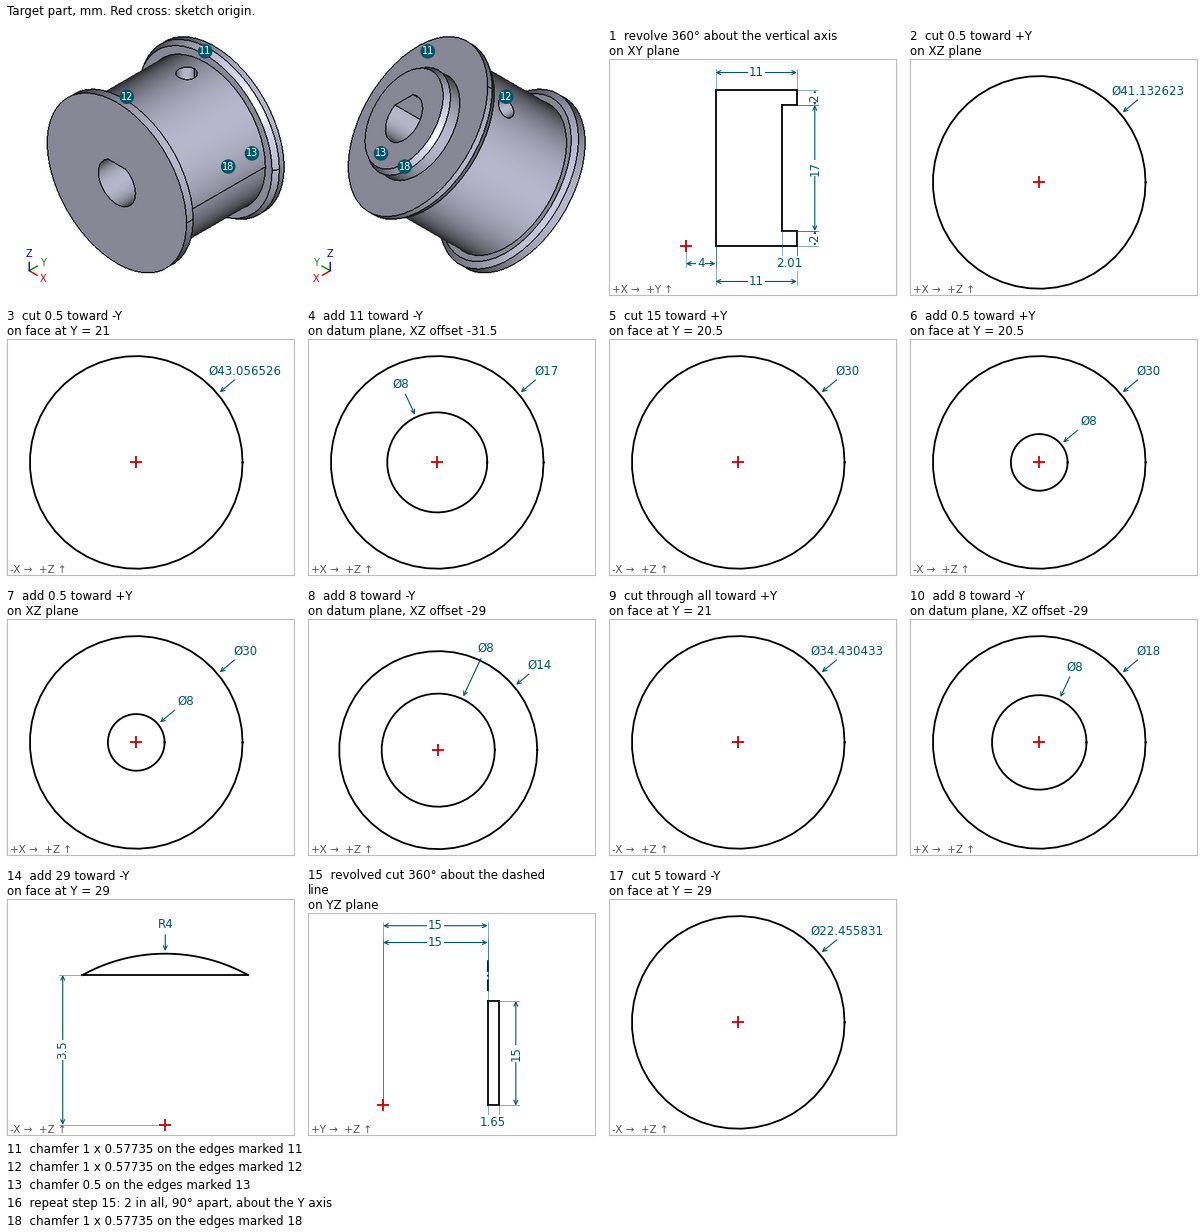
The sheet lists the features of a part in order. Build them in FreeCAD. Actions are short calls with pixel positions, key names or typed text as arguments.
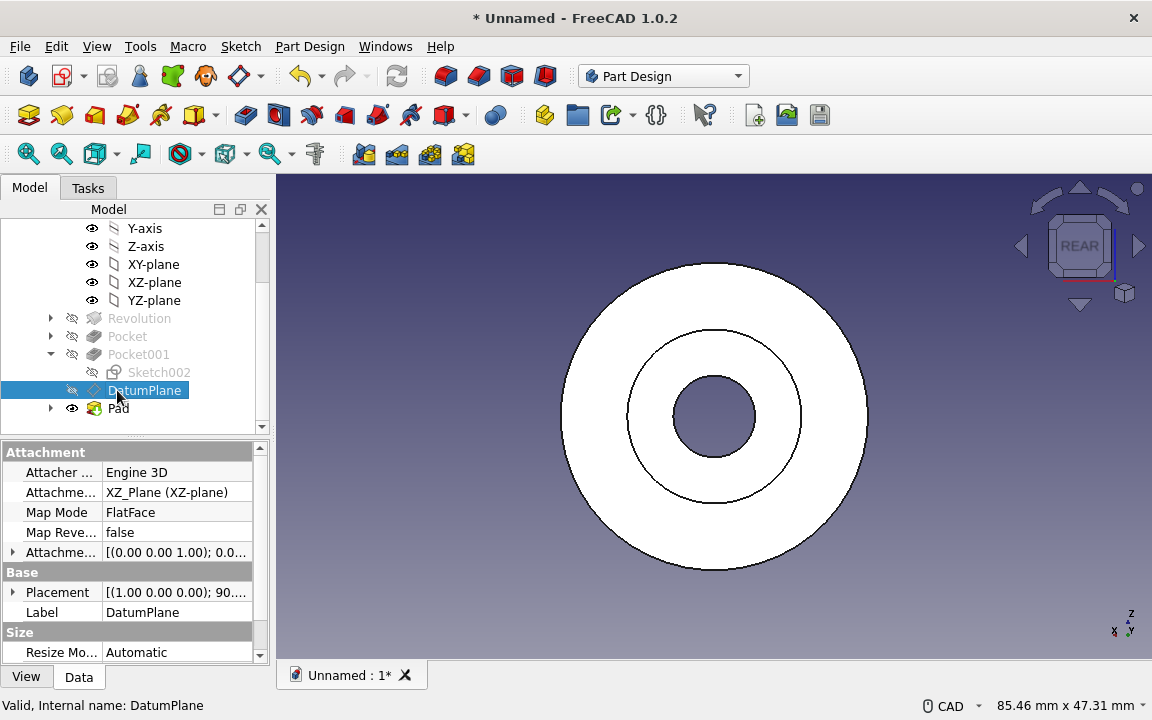
click(802, 328)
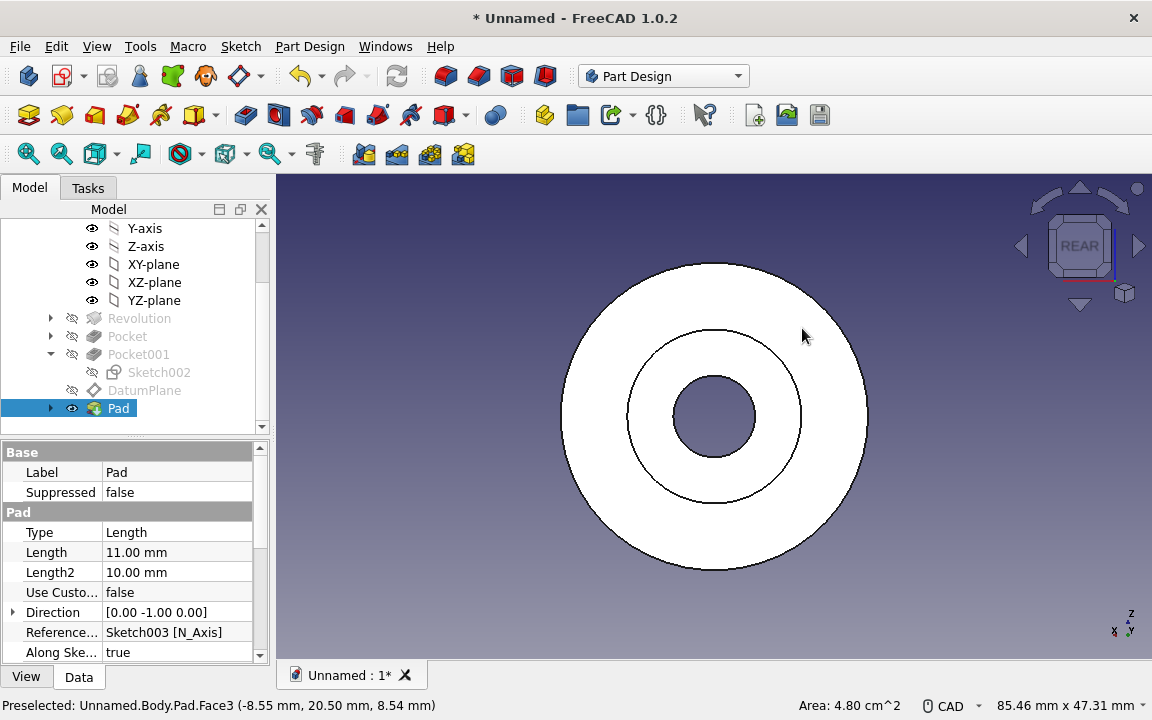
click(62, 76)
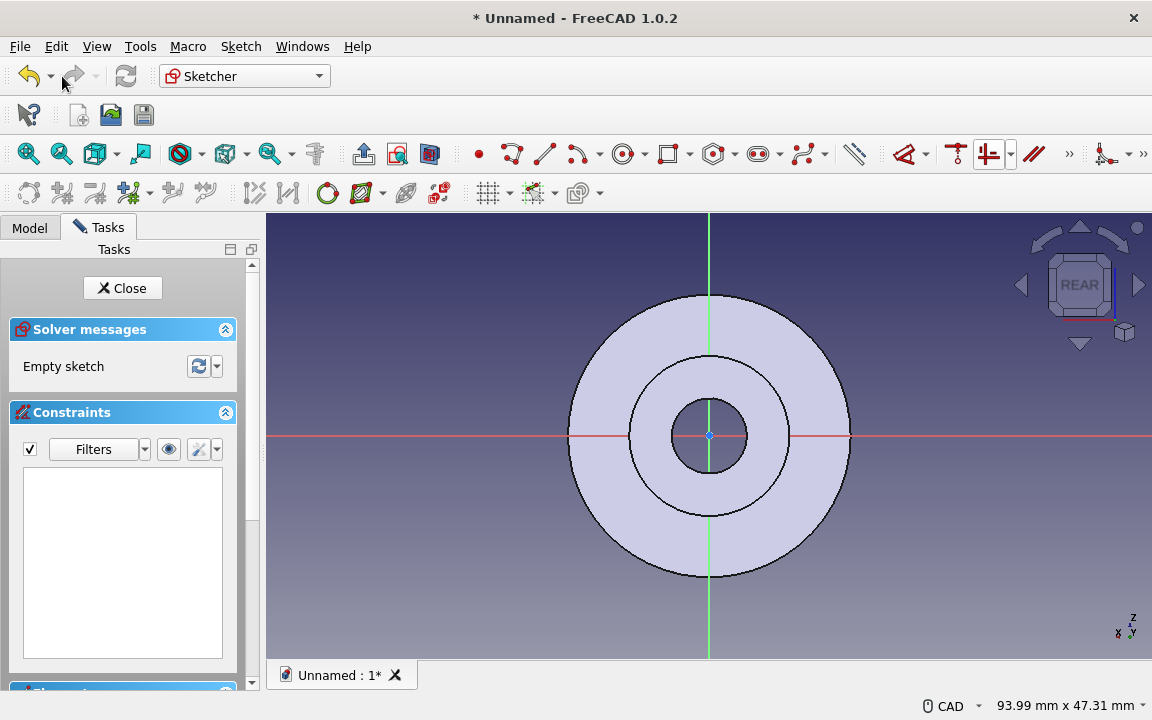
click(622, 154)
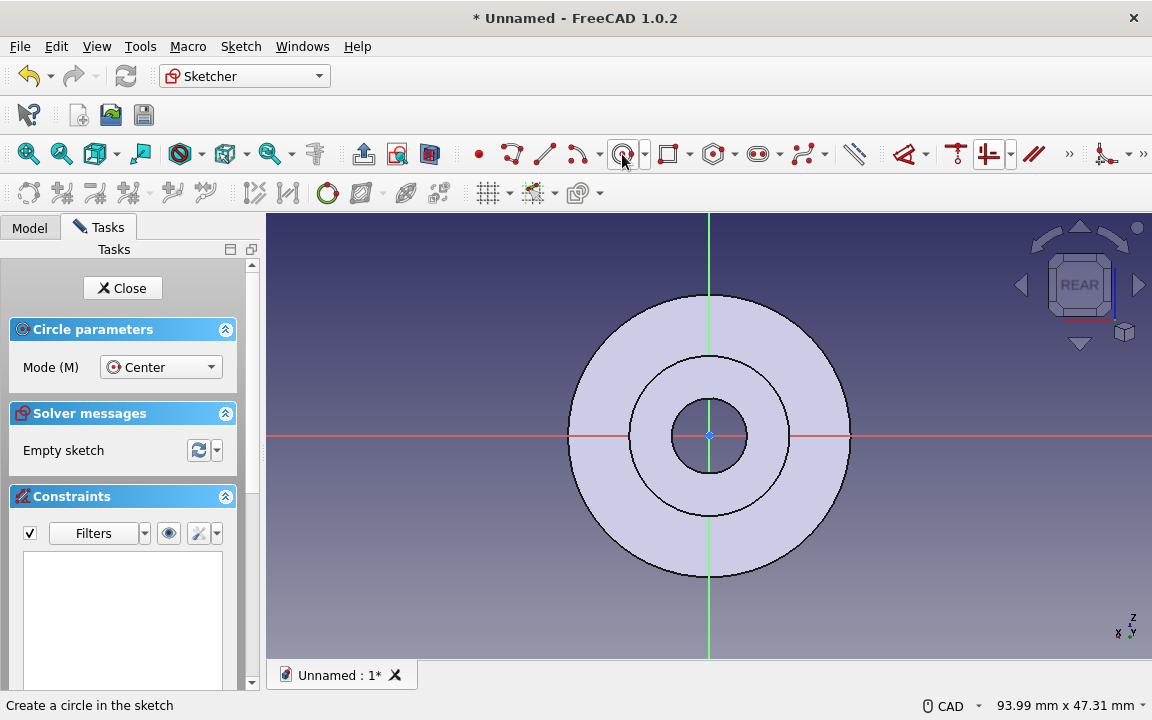
click(709, 436)
move(809, 336)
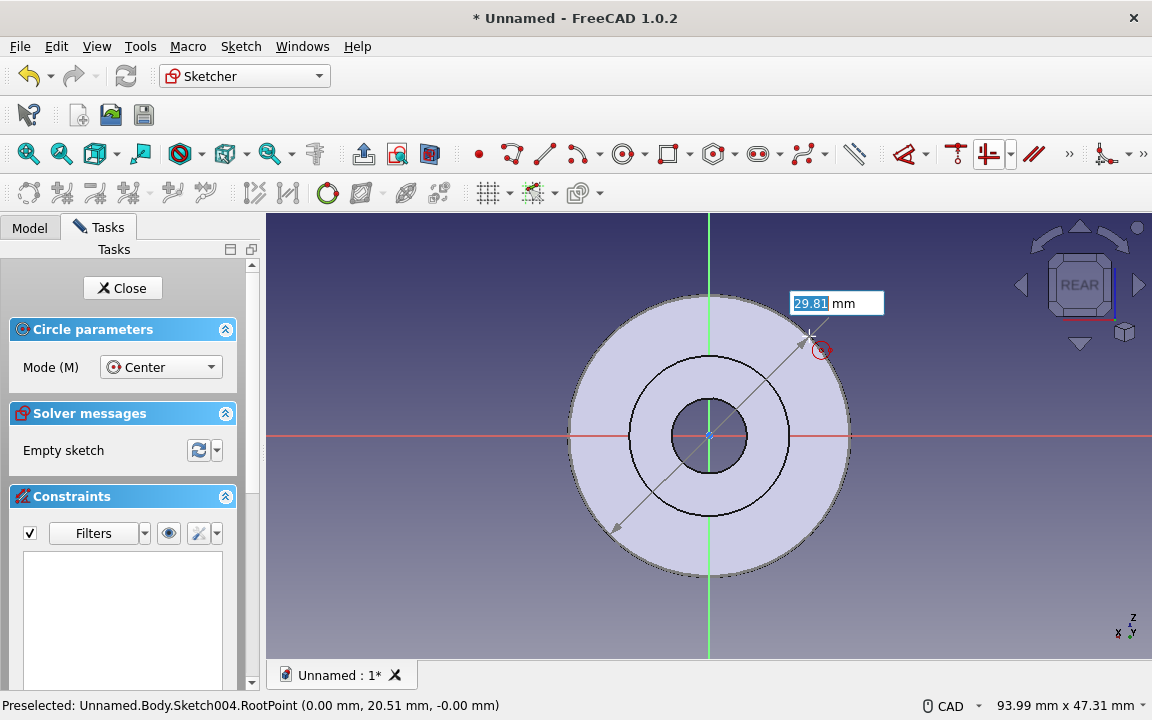
text(30)
key(Return)
key(Escape)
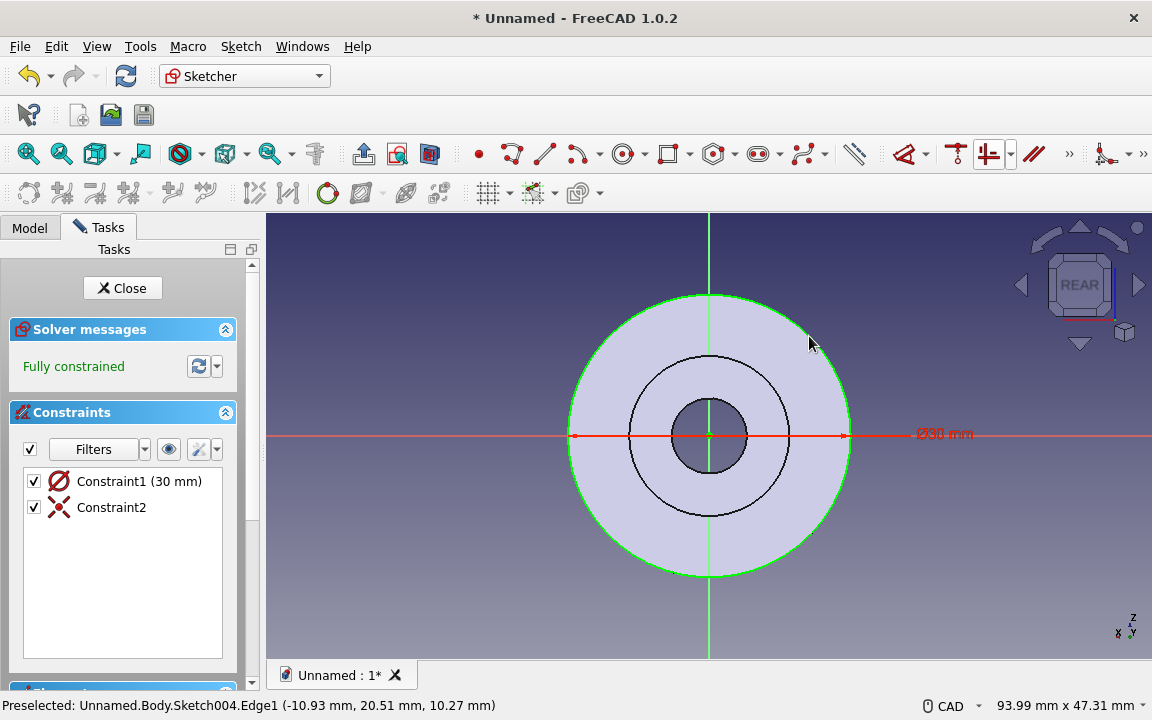
click(123, 288)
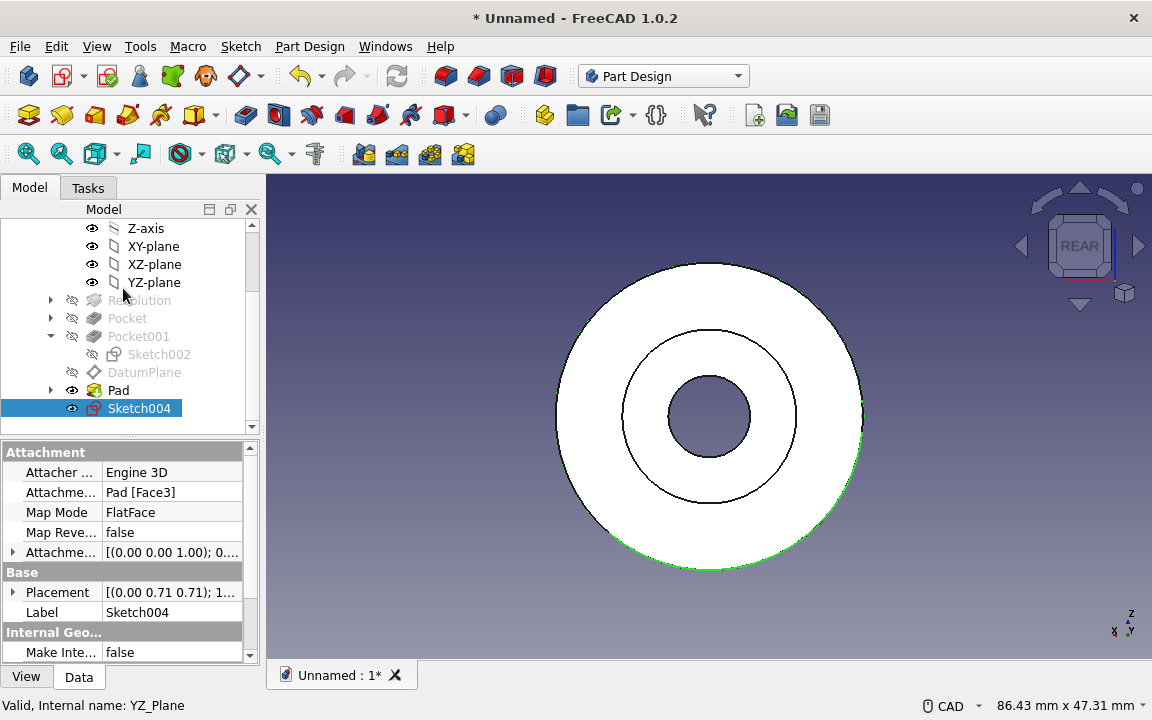
click(246, 116)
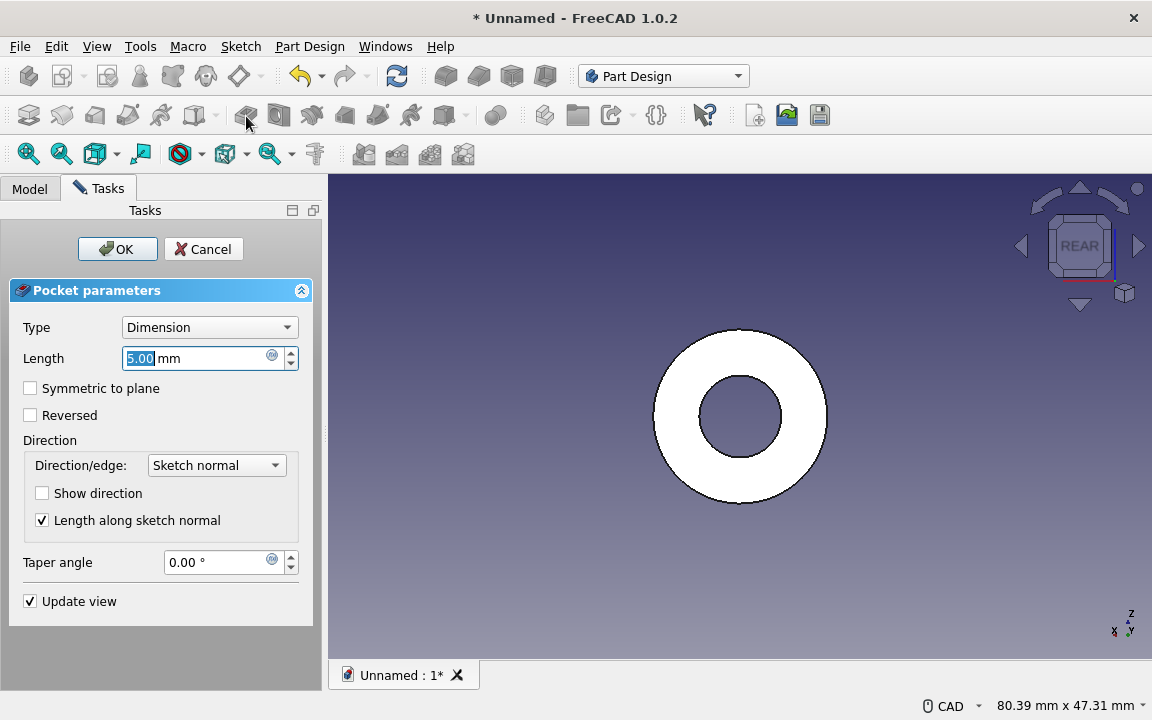
text(15)
key(Tab)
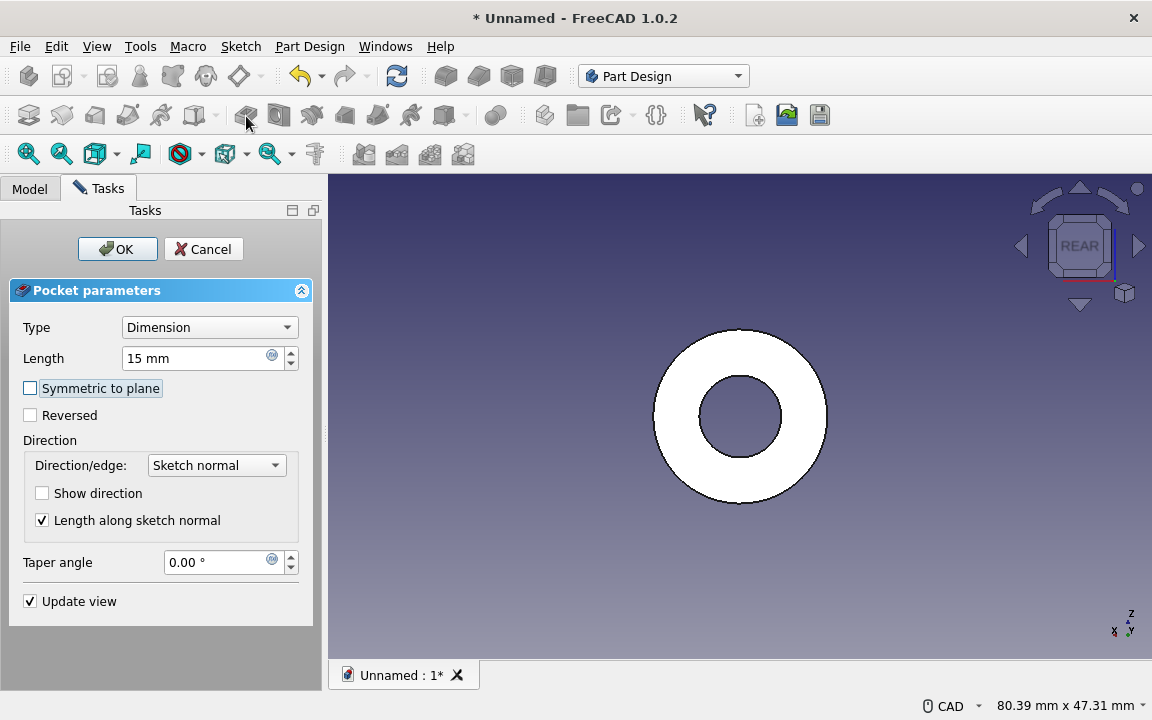
click(31, 415)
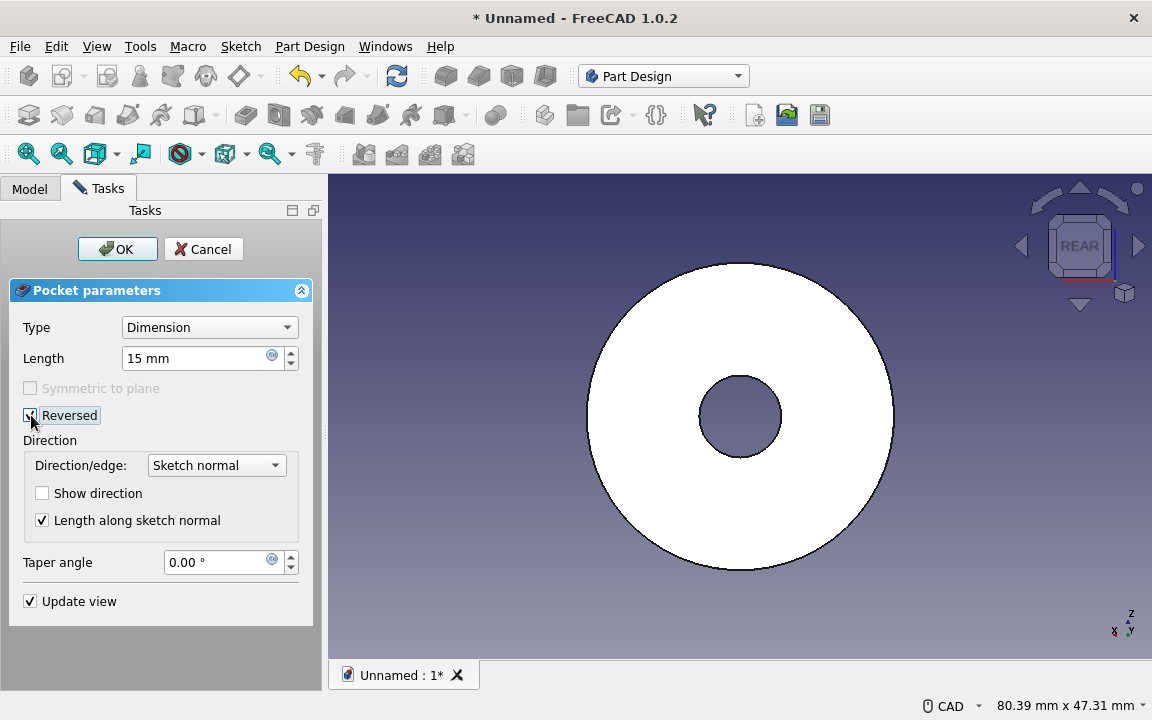
click(118, 249)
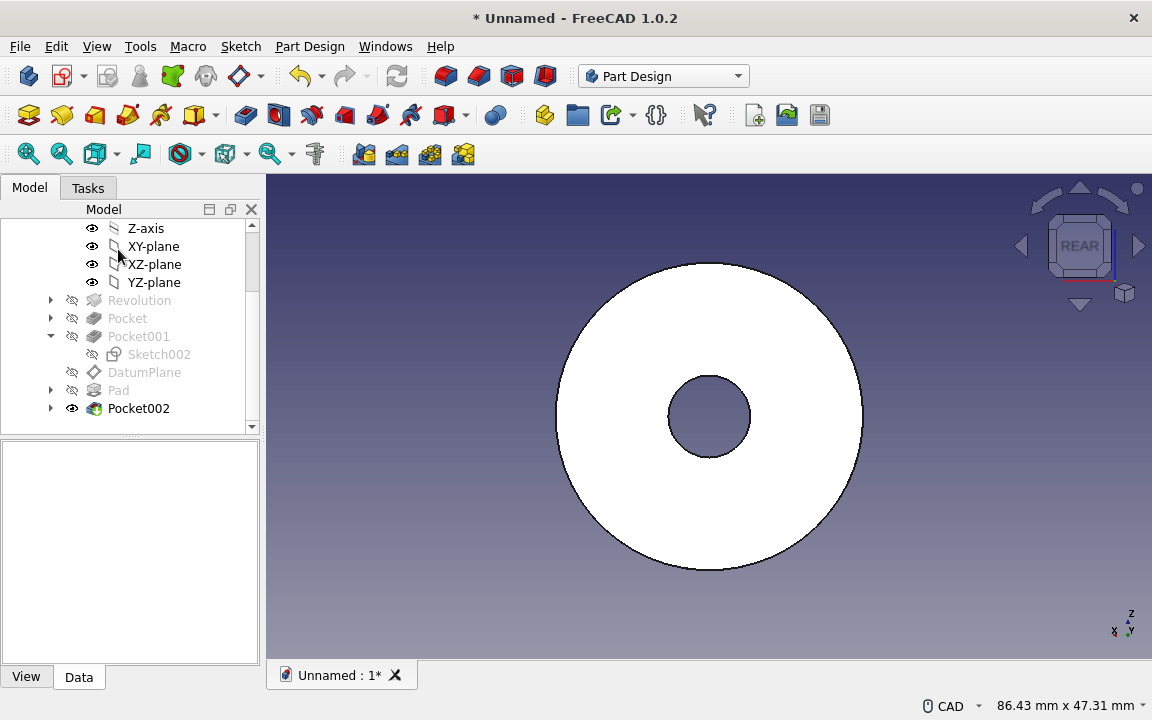
click(797, 372)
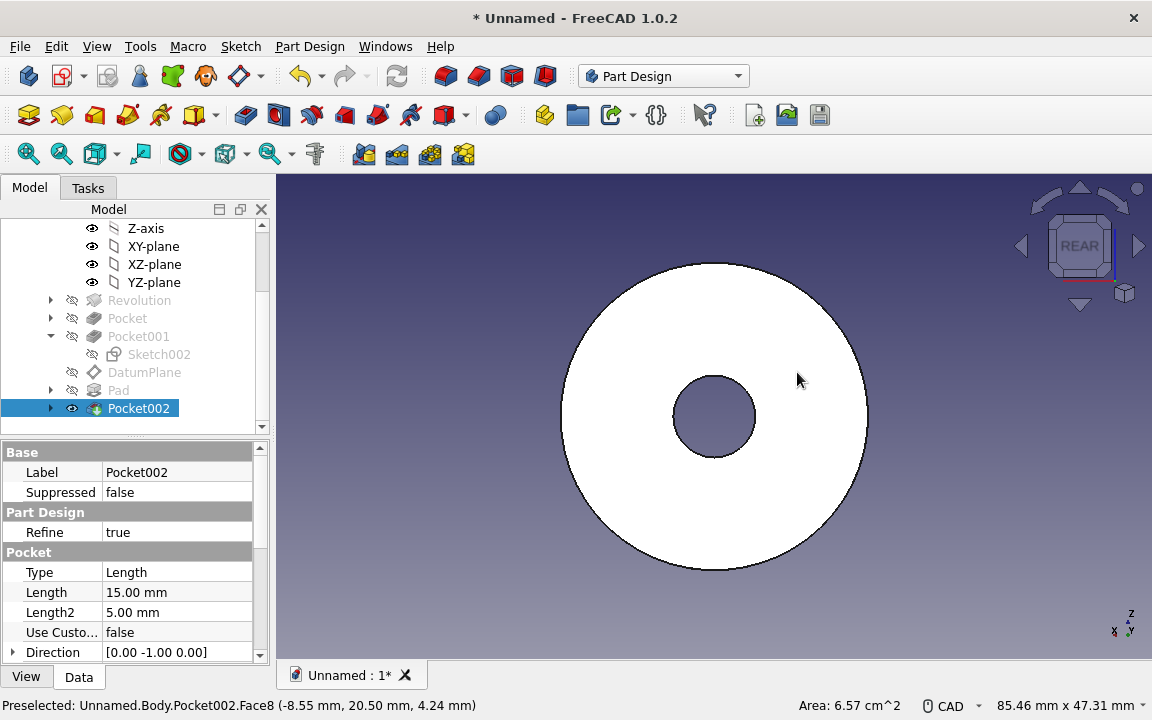
click(62, 76)